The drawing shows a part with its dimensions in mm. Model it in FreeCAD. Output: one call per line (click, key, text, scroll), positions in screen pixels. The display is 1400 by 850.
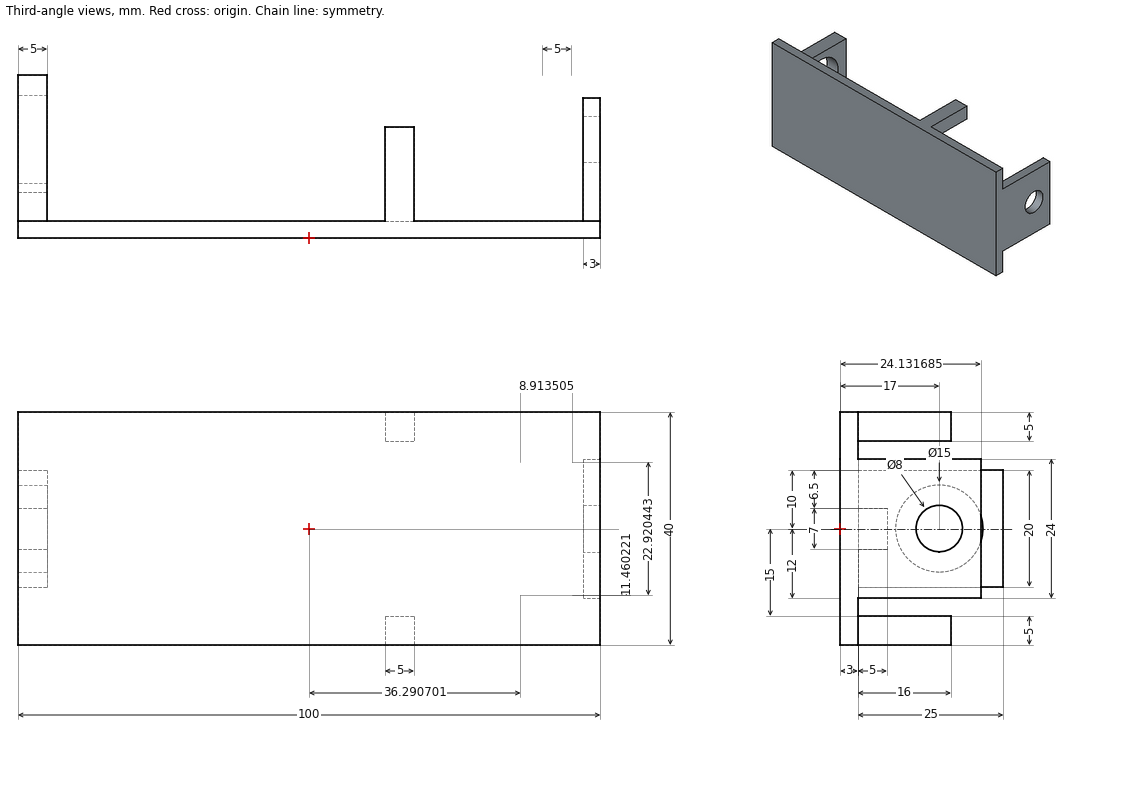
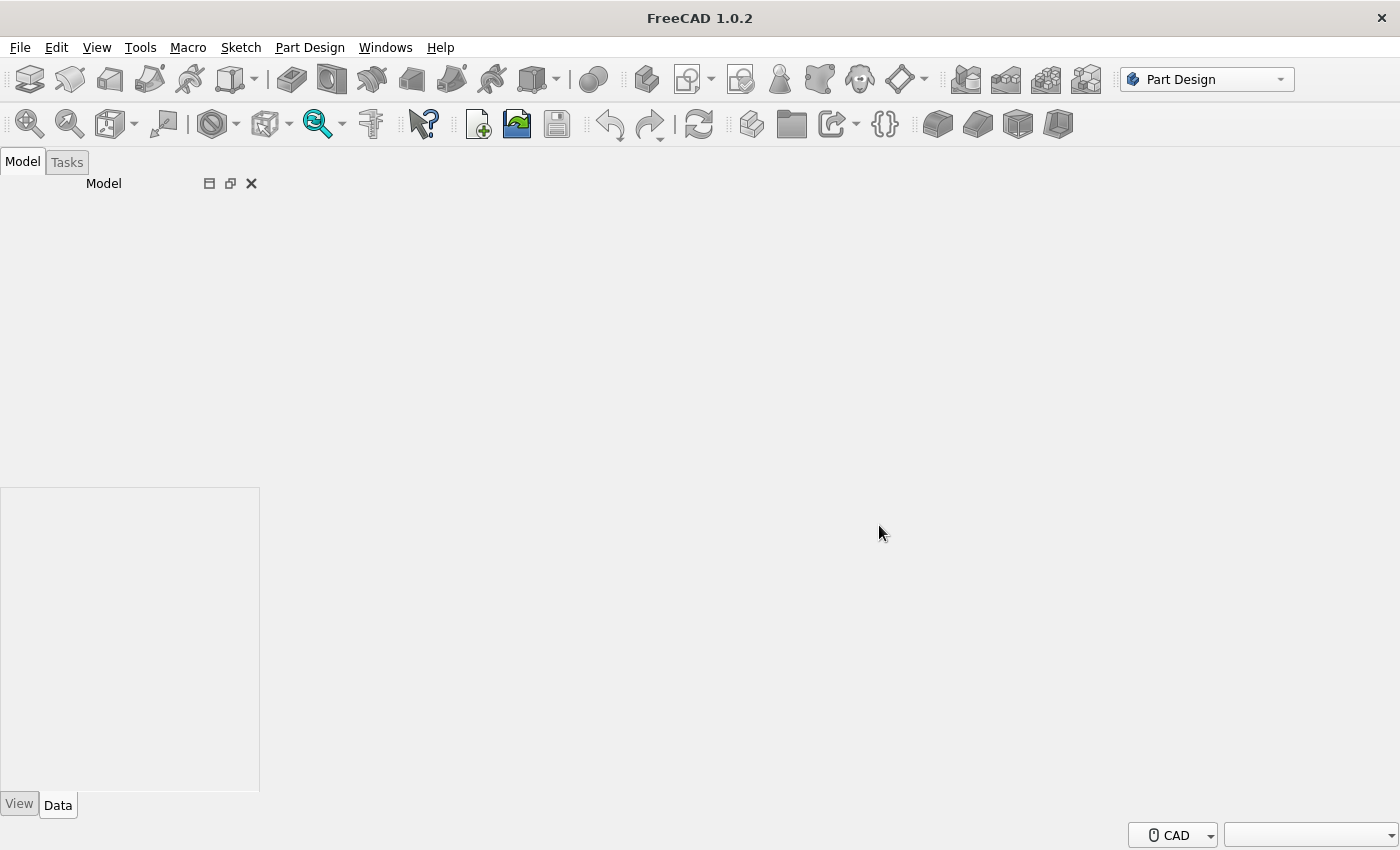
key(ctrl+n)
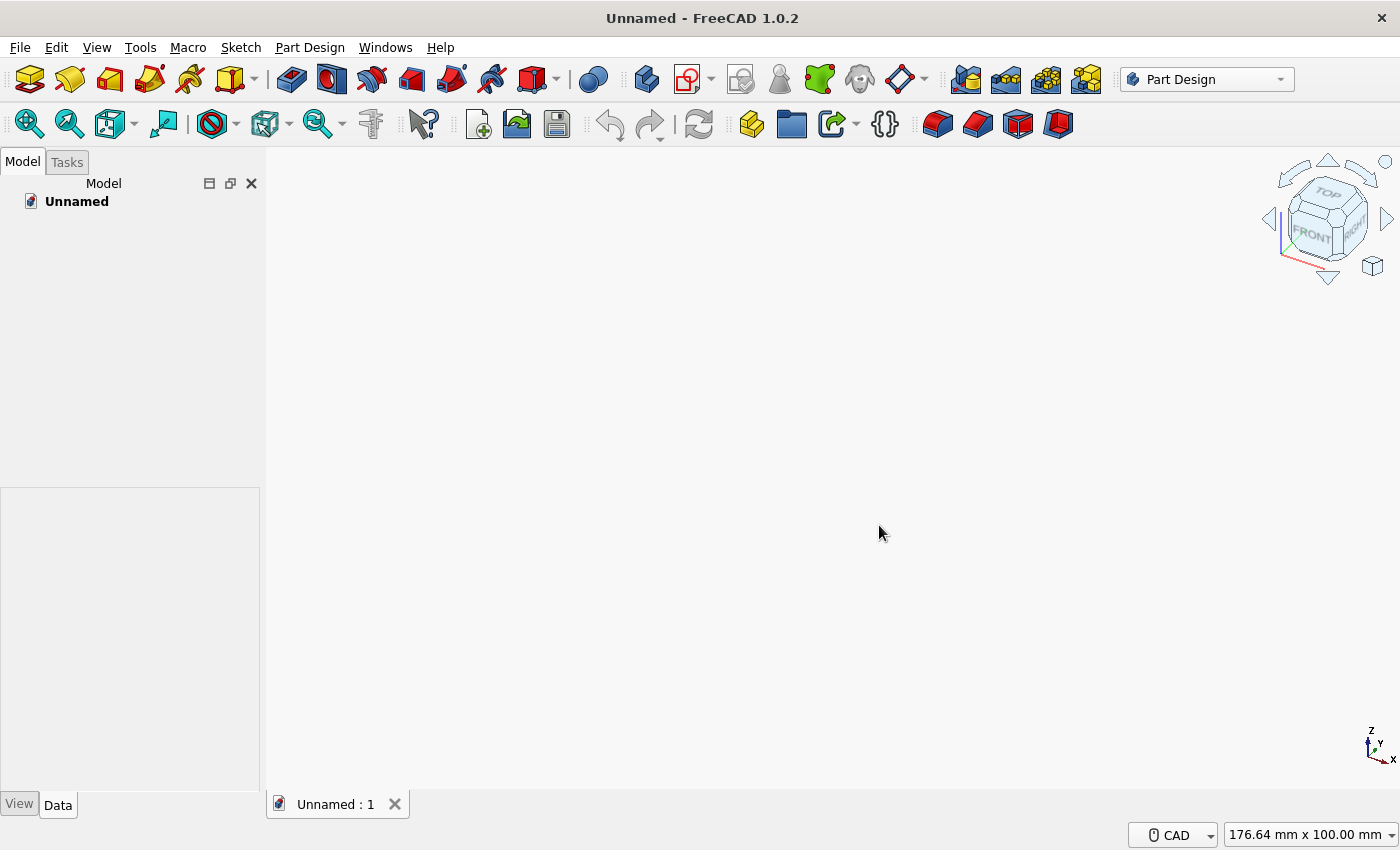
click(688, 80)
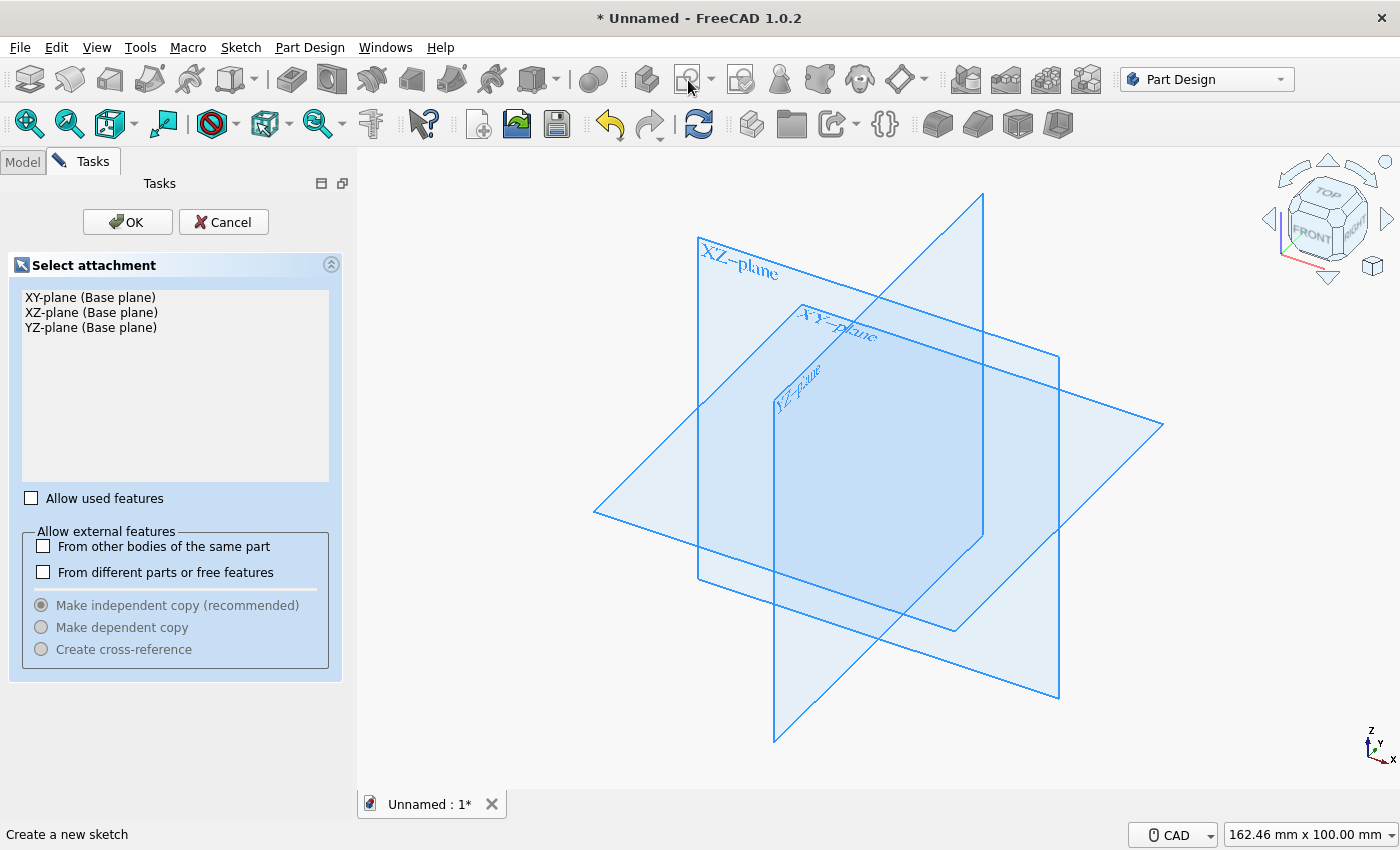
click(82, 312)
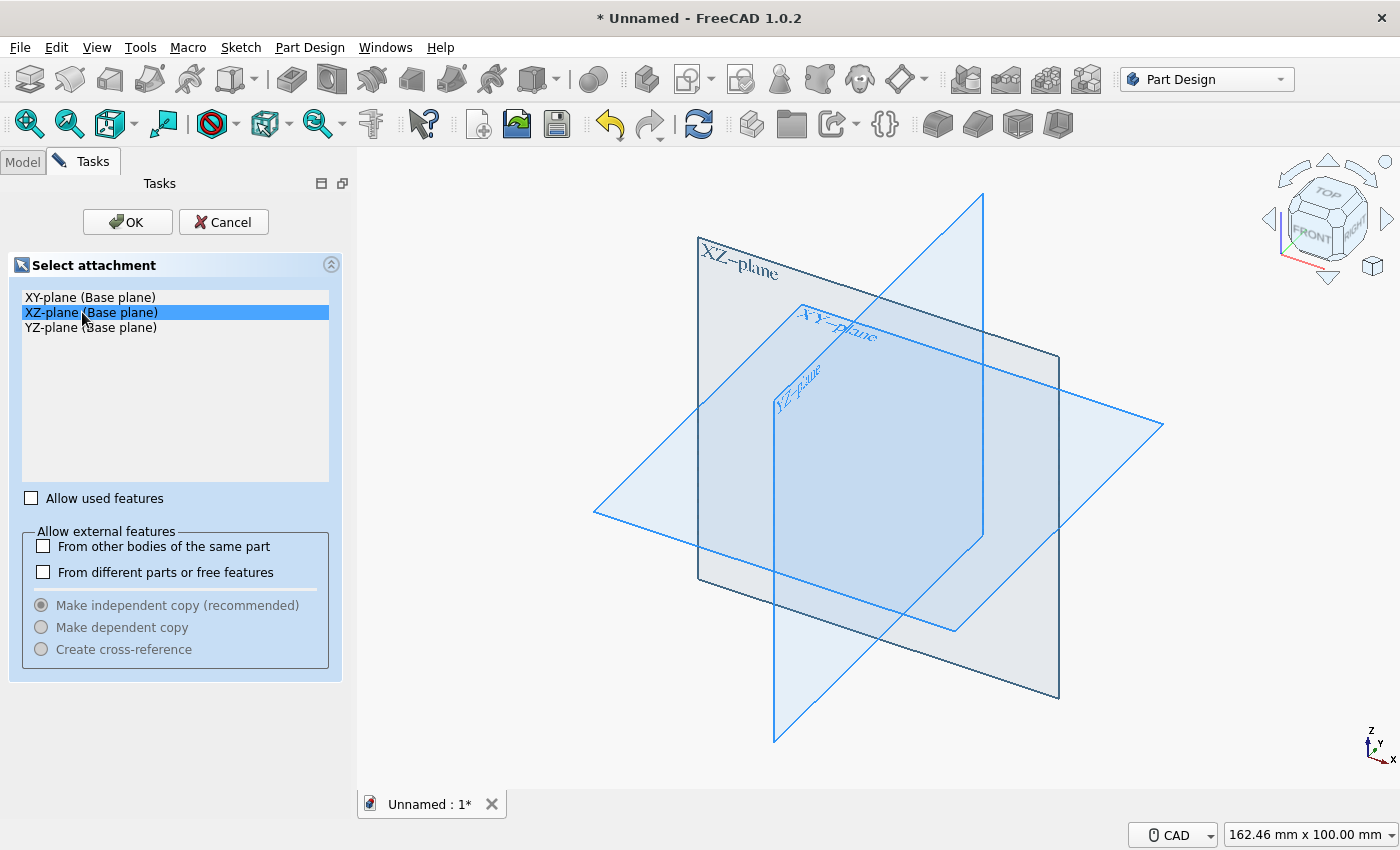
click(128, 222)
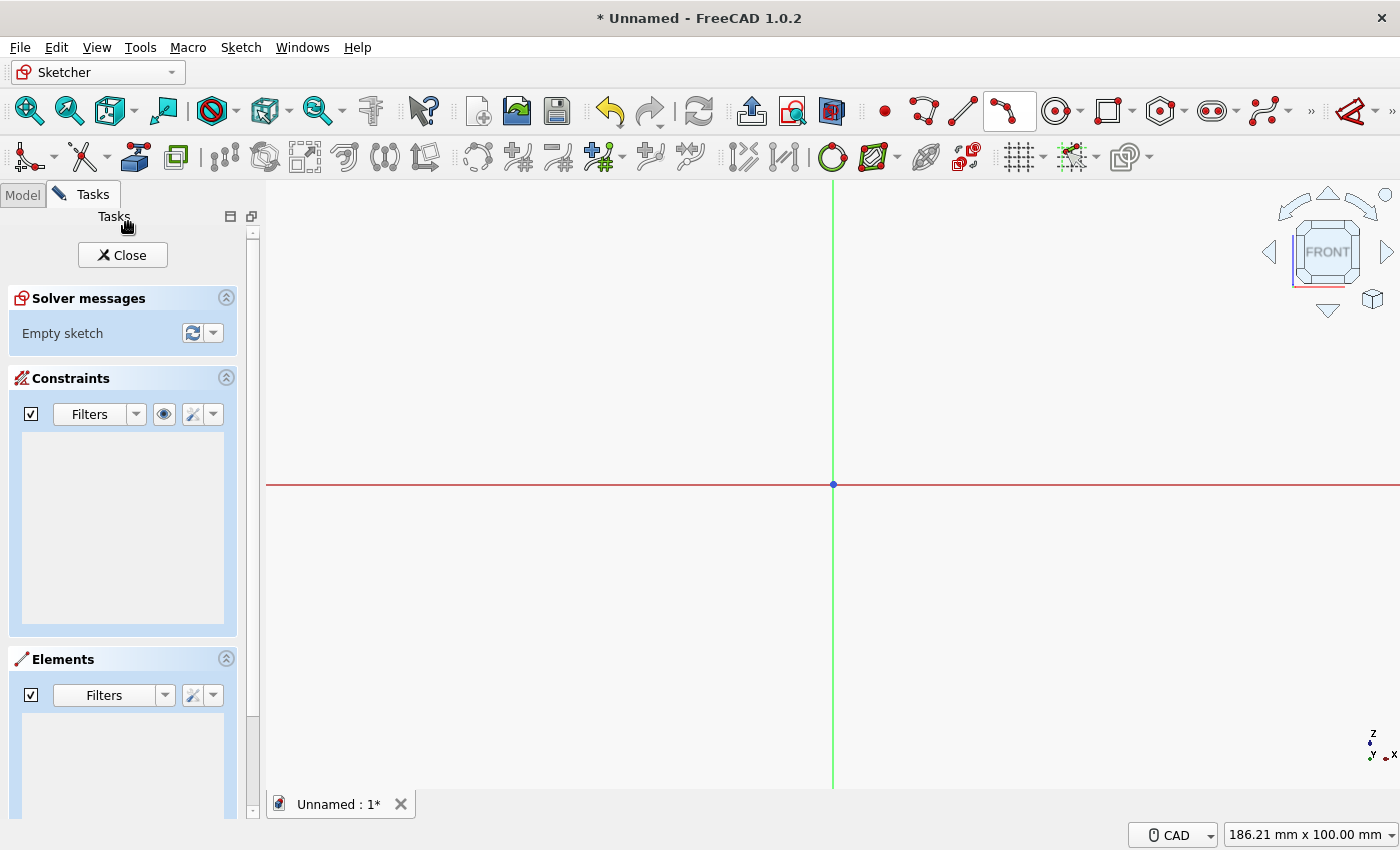
key(g)
key(v)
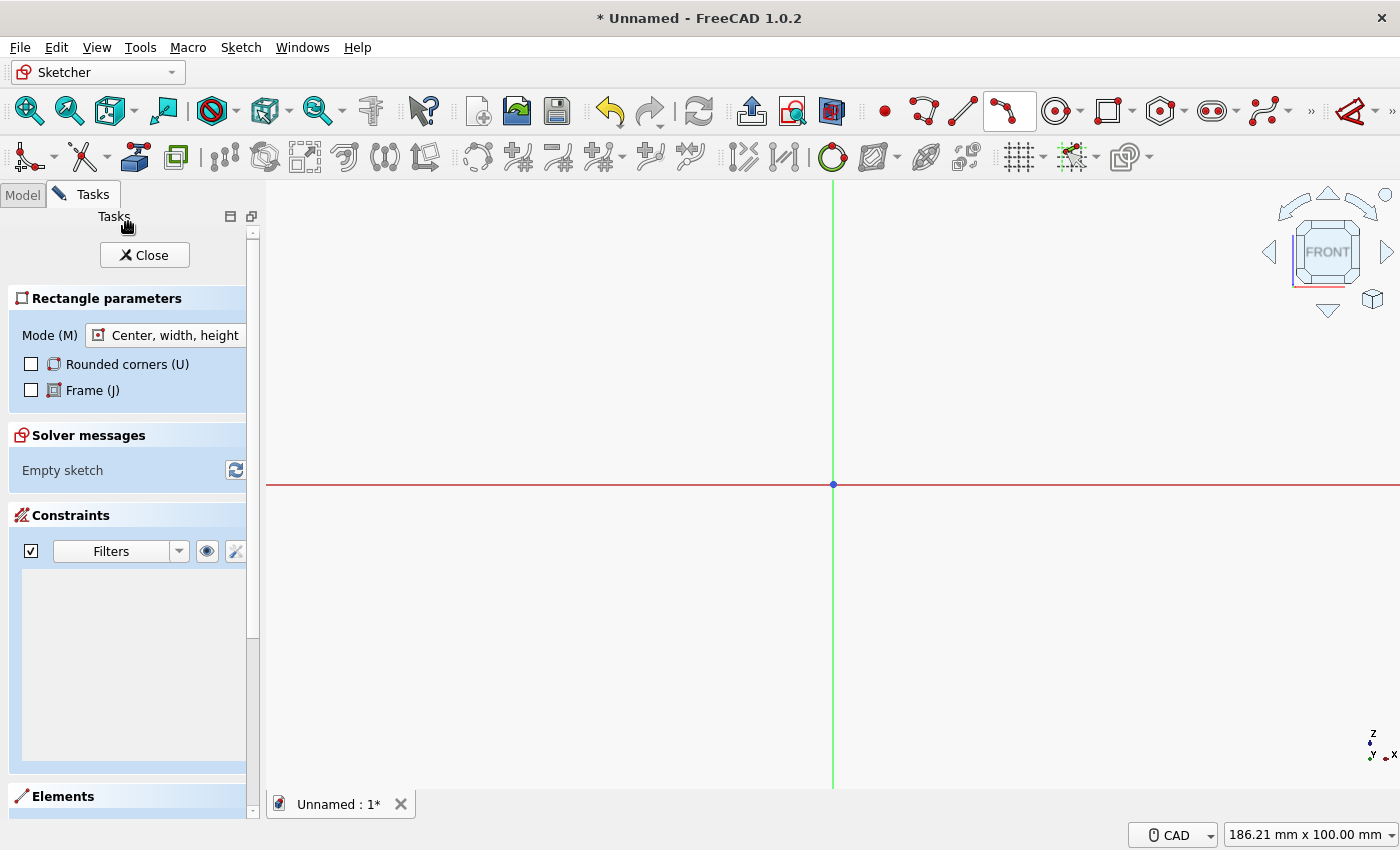
click(833, 484)
move(1138, 363)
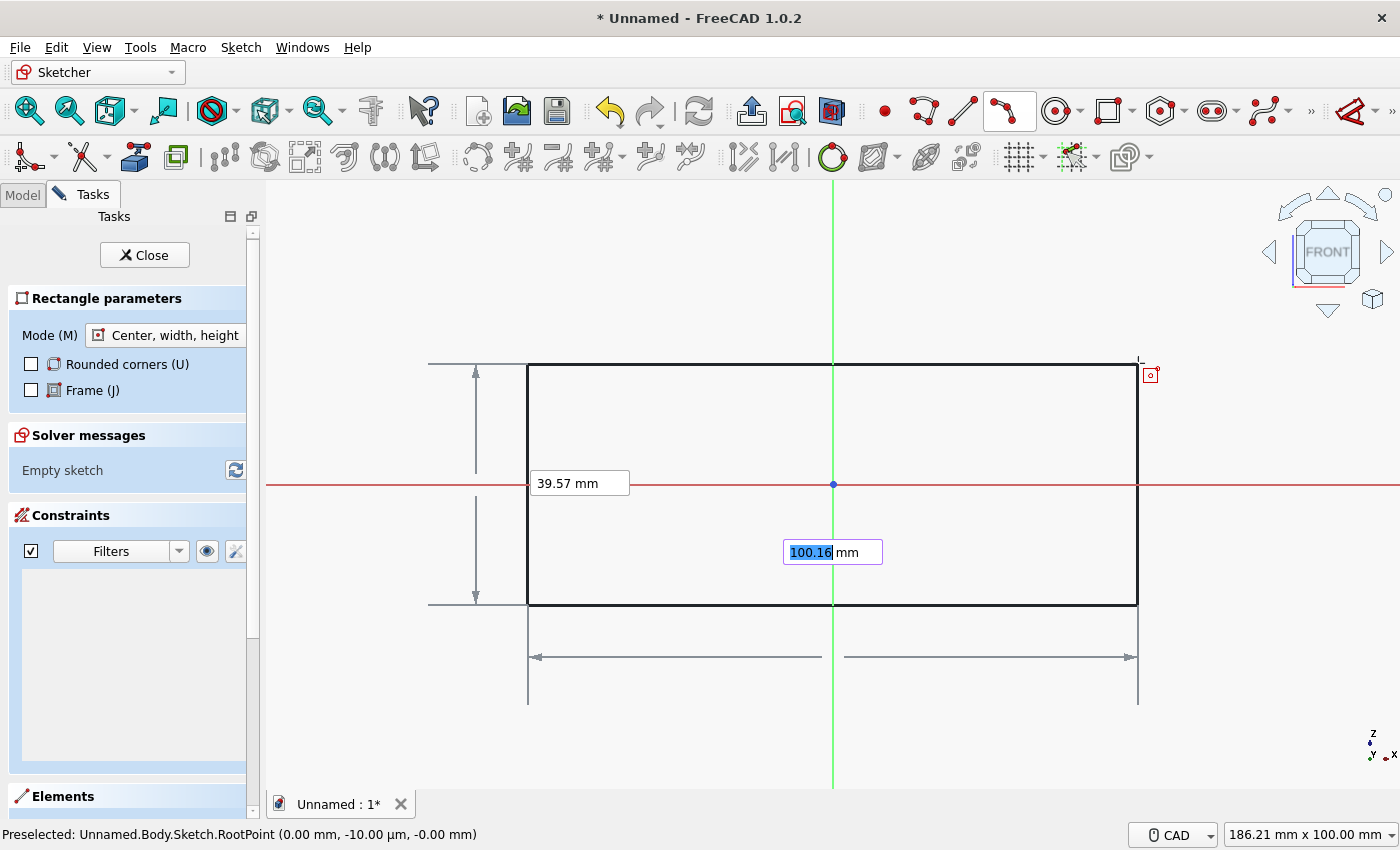
text(100)
key(Tab)
text(40)
key(Return)
key(Escape)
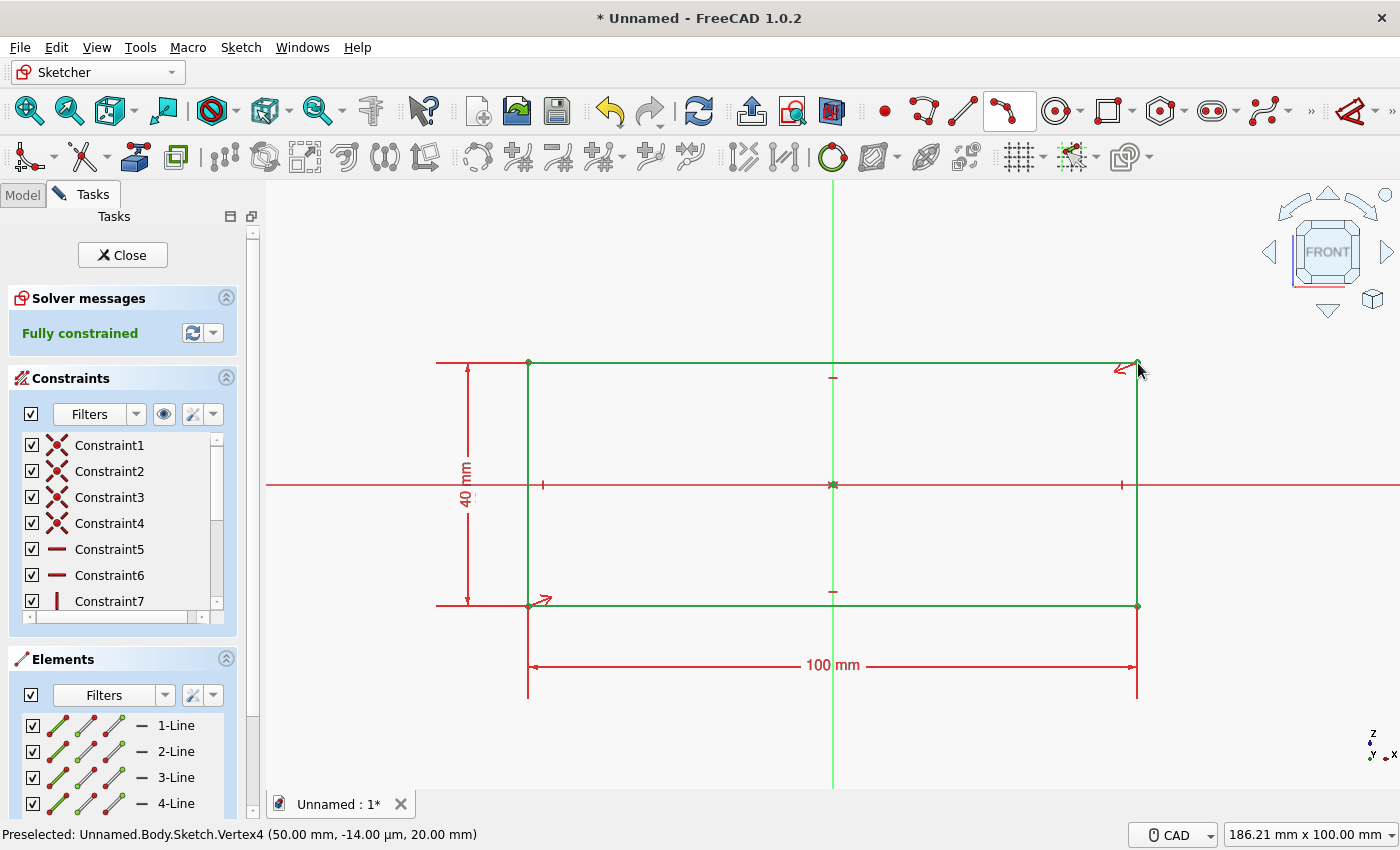
click(123, 255)